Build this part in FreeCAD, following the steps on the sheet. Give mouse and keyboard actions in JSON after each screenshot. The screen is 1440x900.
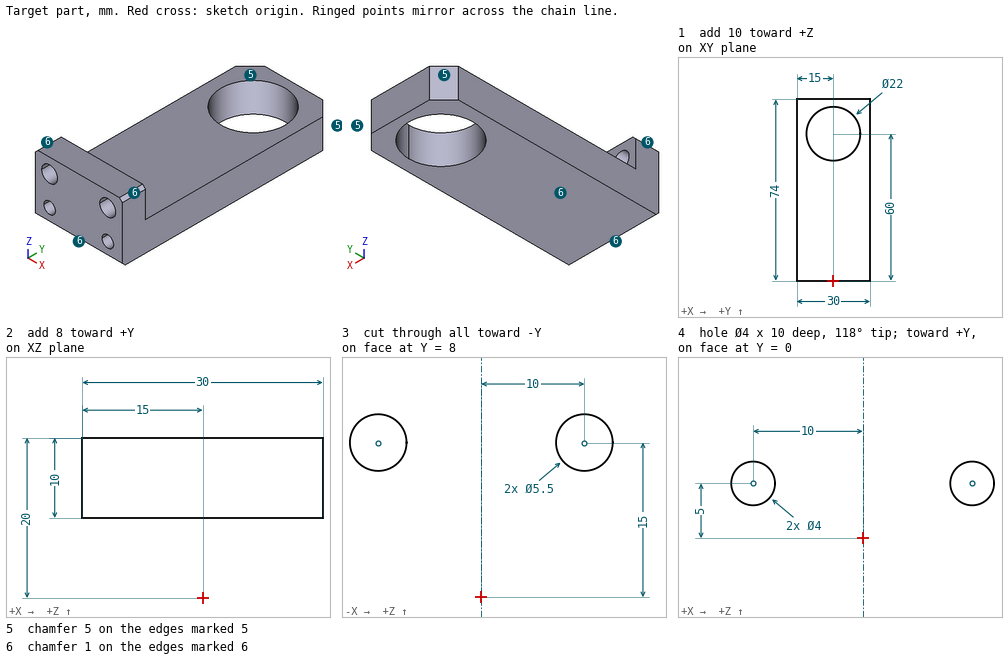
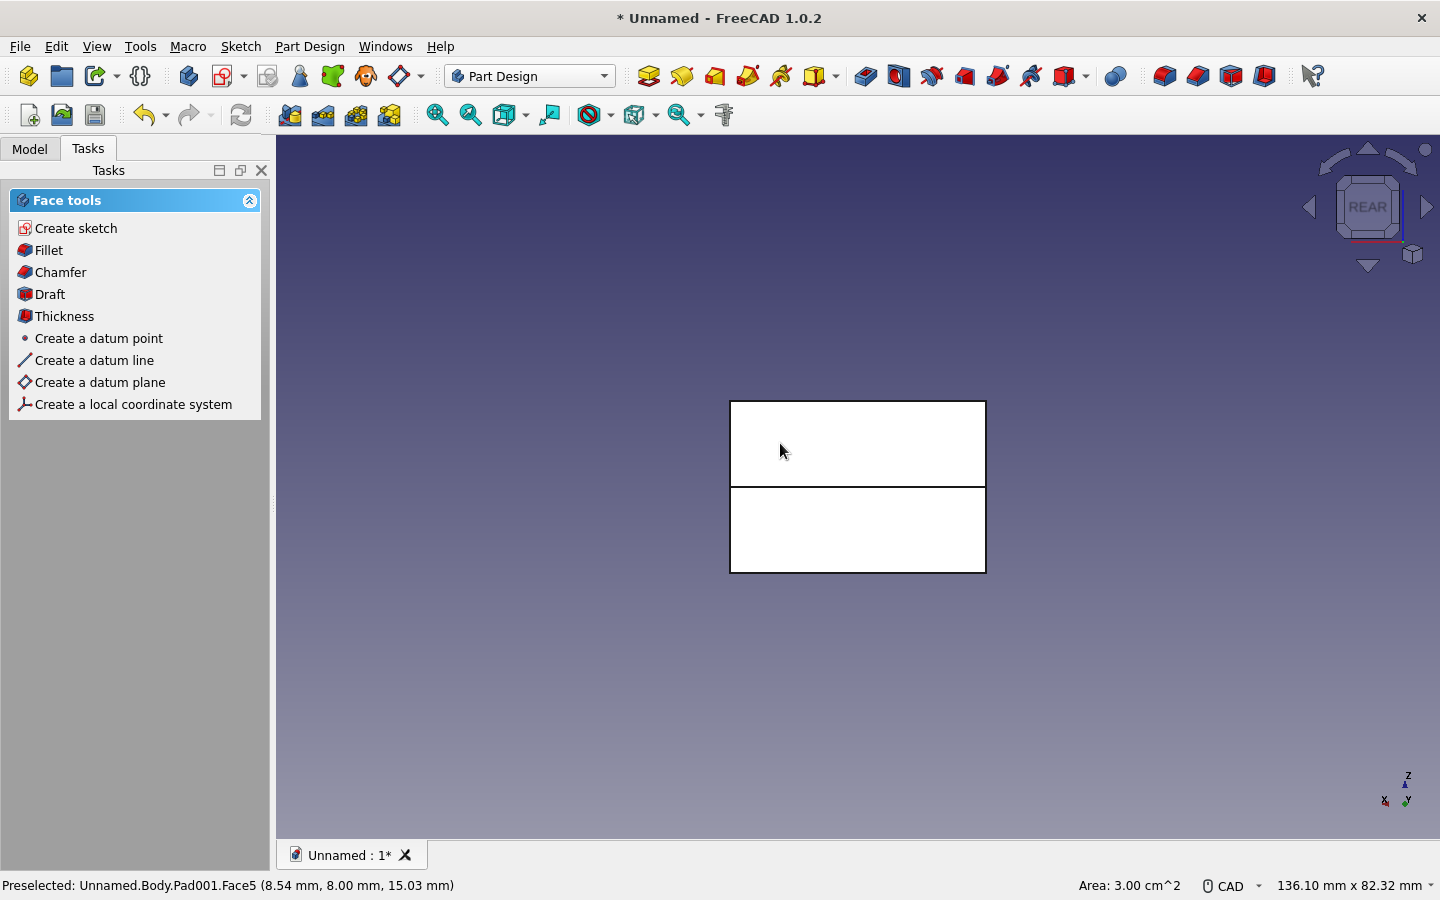
{"action": "left_click", "coordinate": [222, 76]}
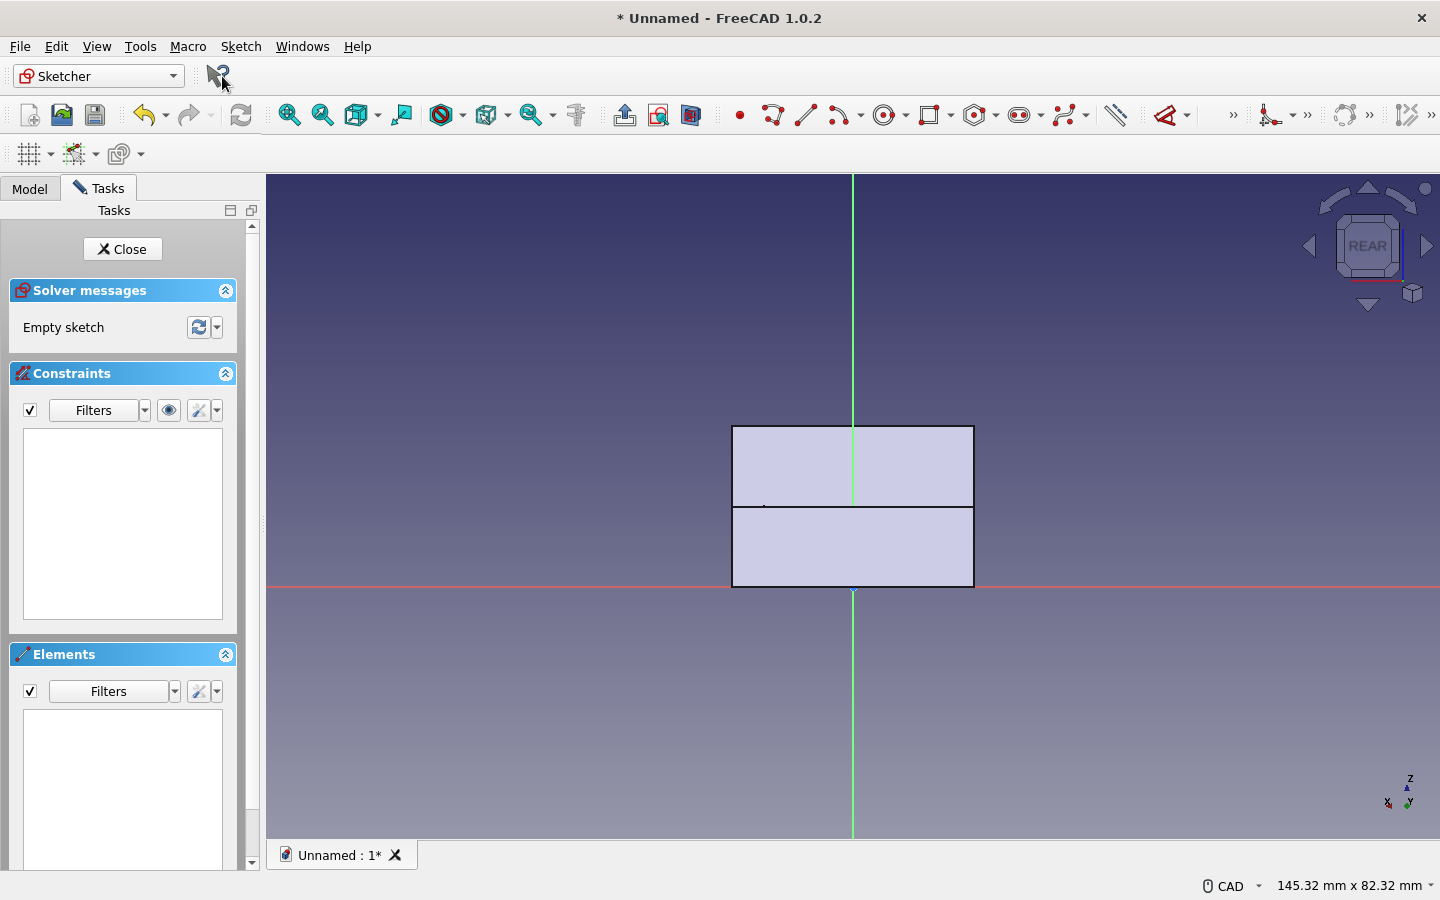
{"action": "left_click", "coordinate": [691, 116]}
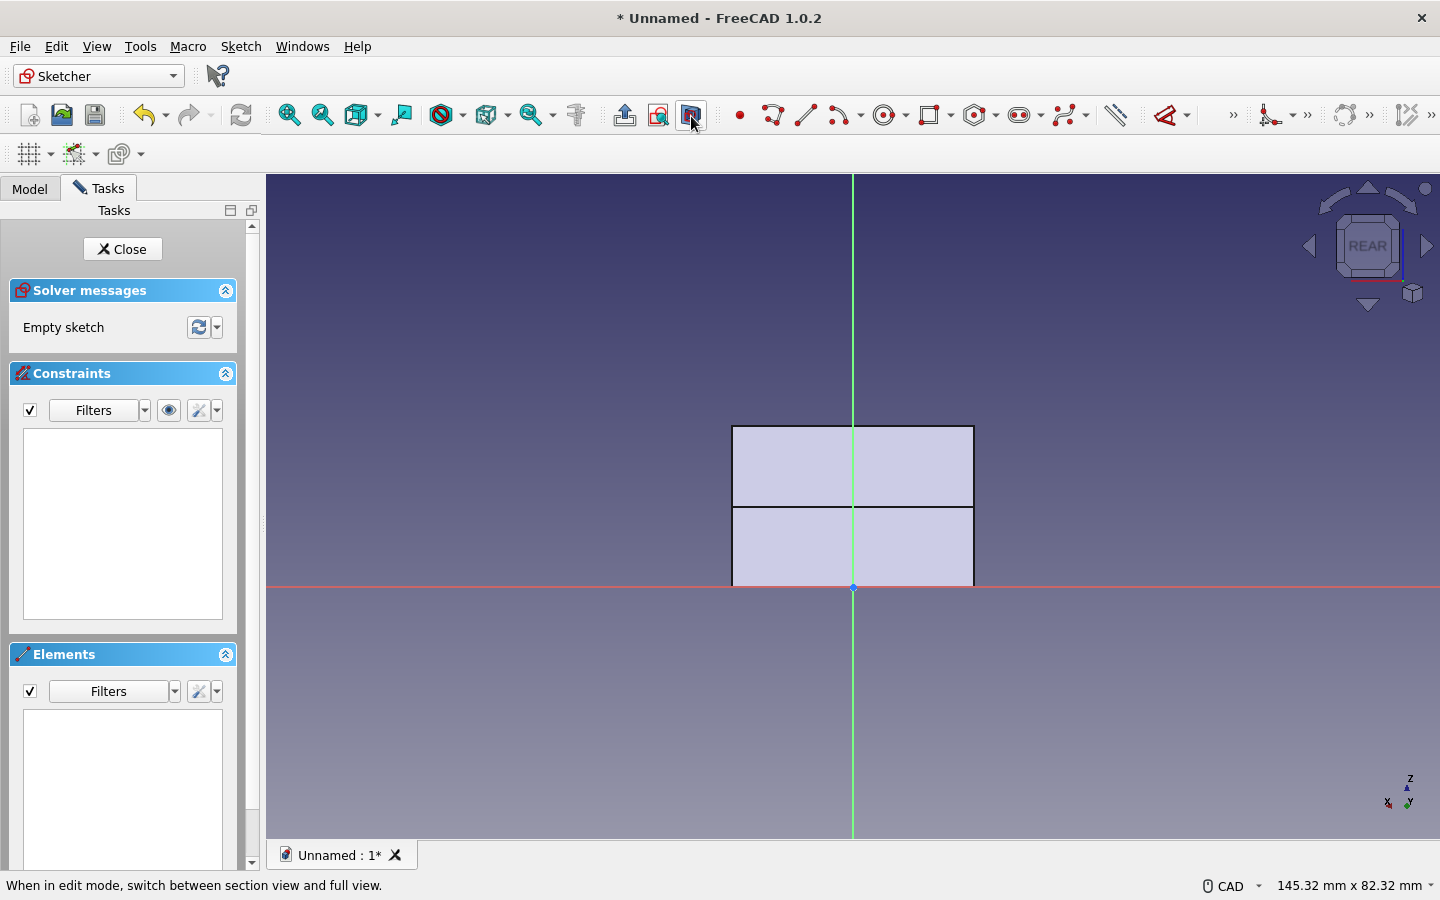
{"action": "scroll", "coordinate": [893, 521], "scroll_direction": "up", "scroll_amount": 5}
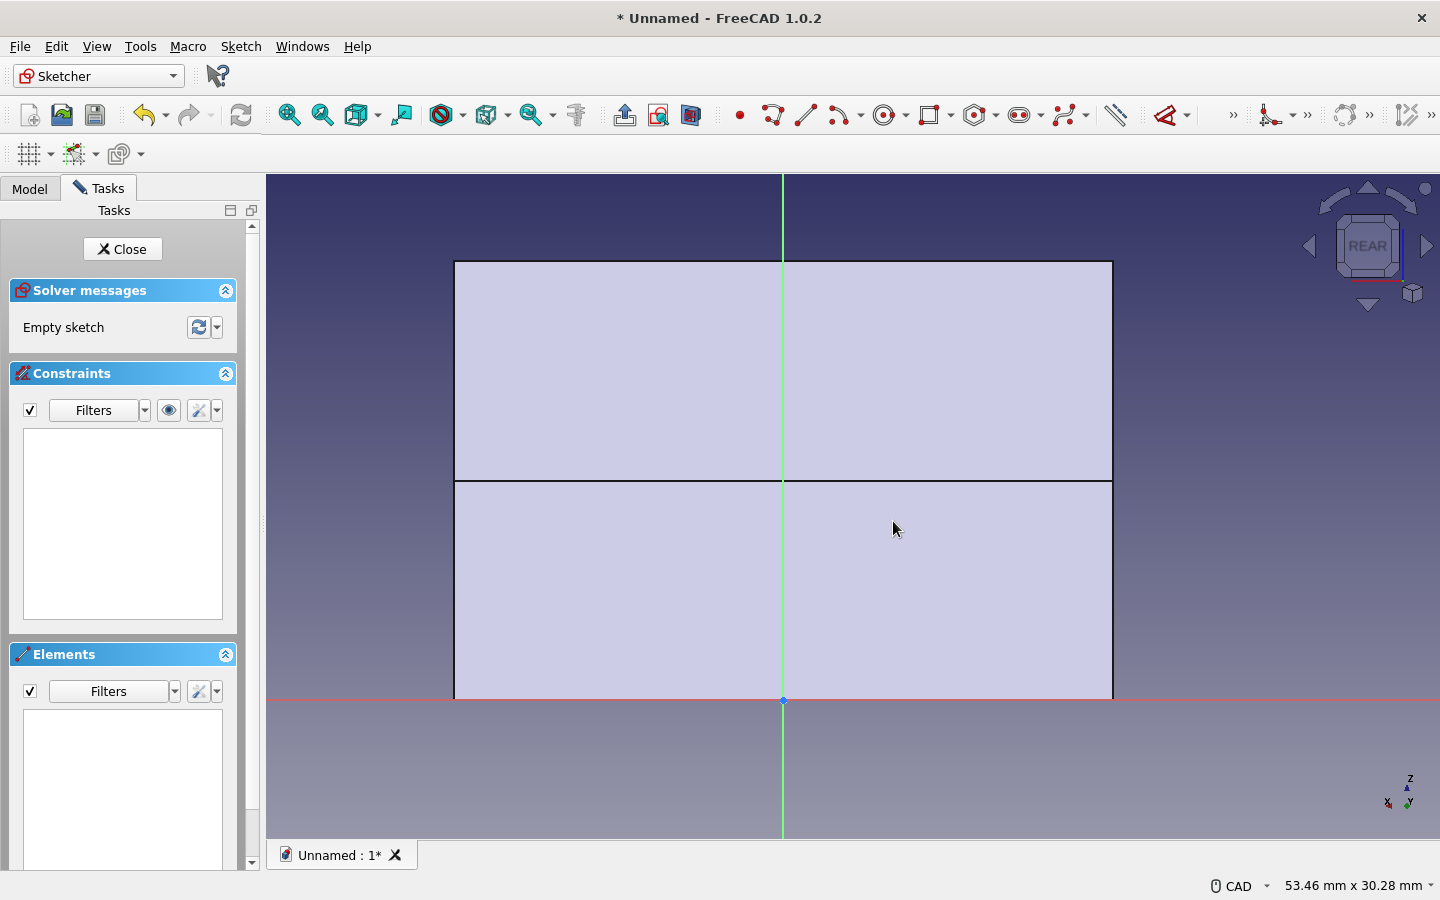
{"action": "left_click", "coordinate": [884, 116]}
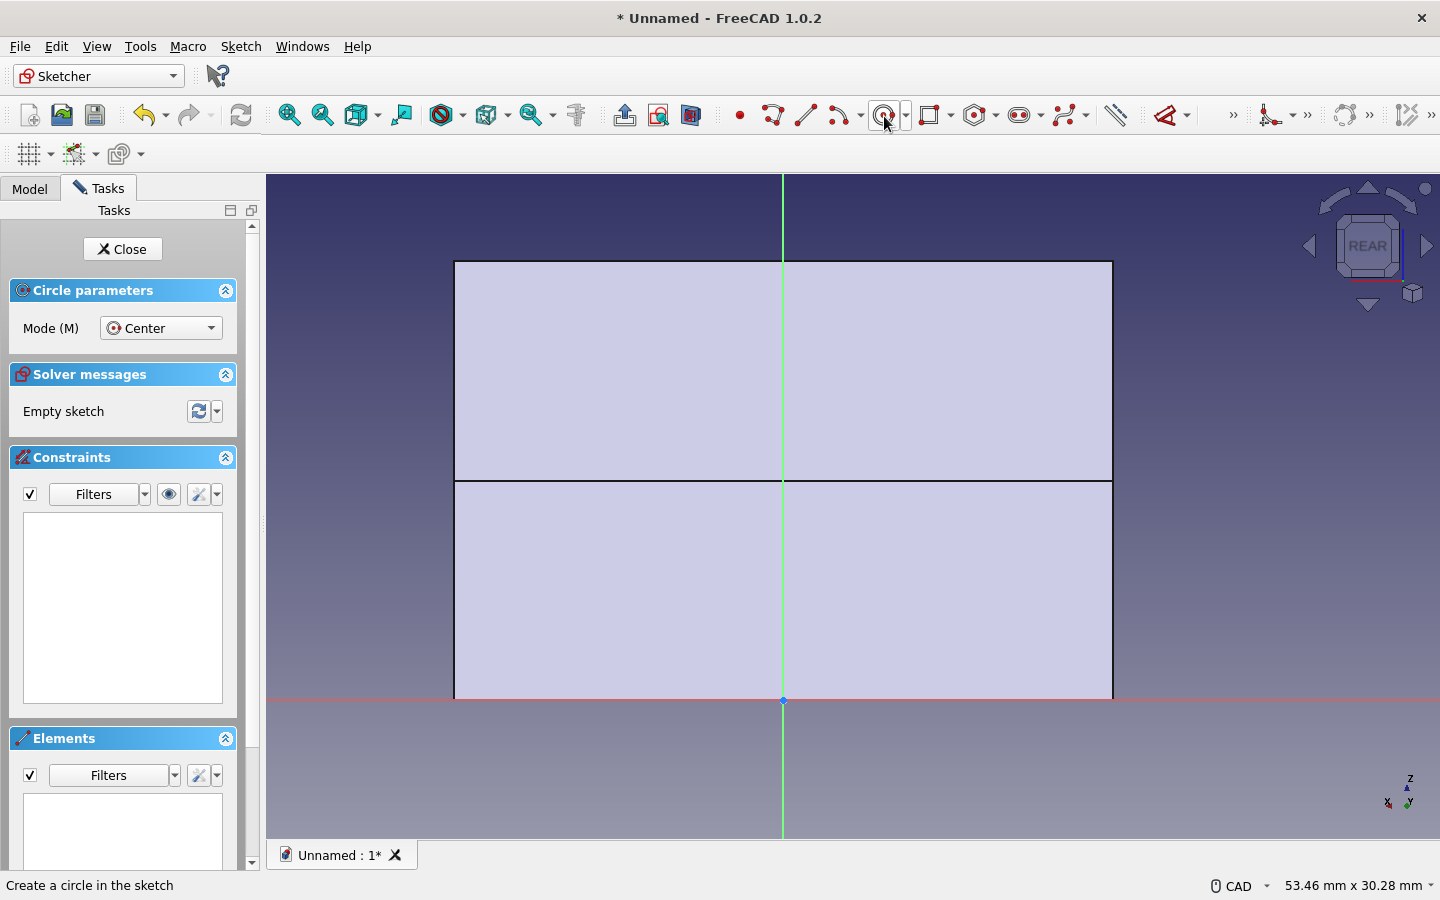
{"action": "left_click", "coordinate": [1003, 371]}
{"action": "left_click", "coordinate": [1046, 328]}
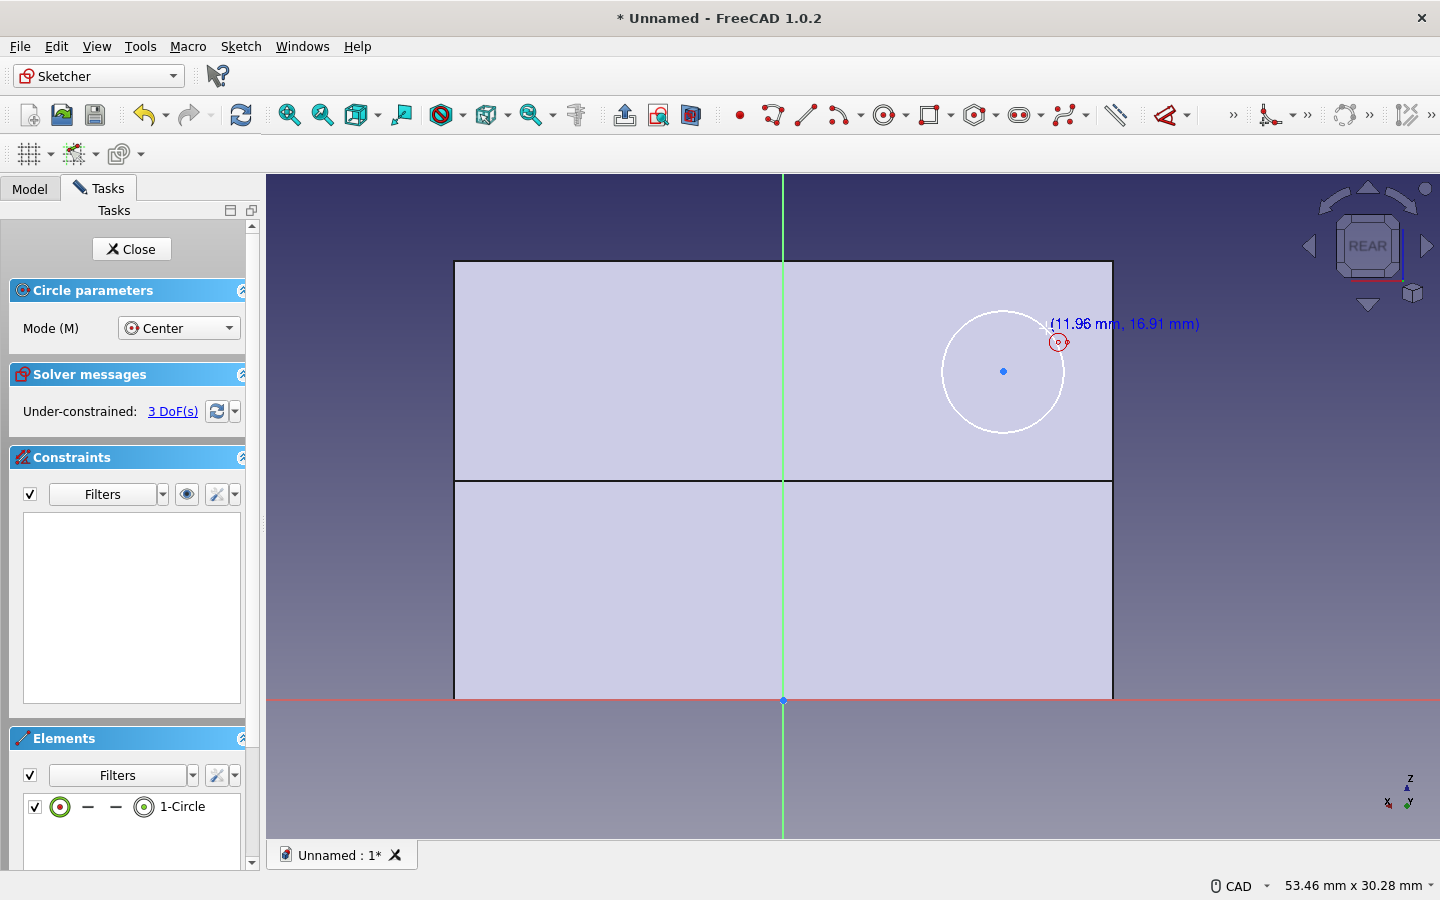
{"action": "left_click", "coordinate": [564, 371]}
{"action": "left_click", "coordinate": [606, 328]}
{"action": "key", "text": "Escape"}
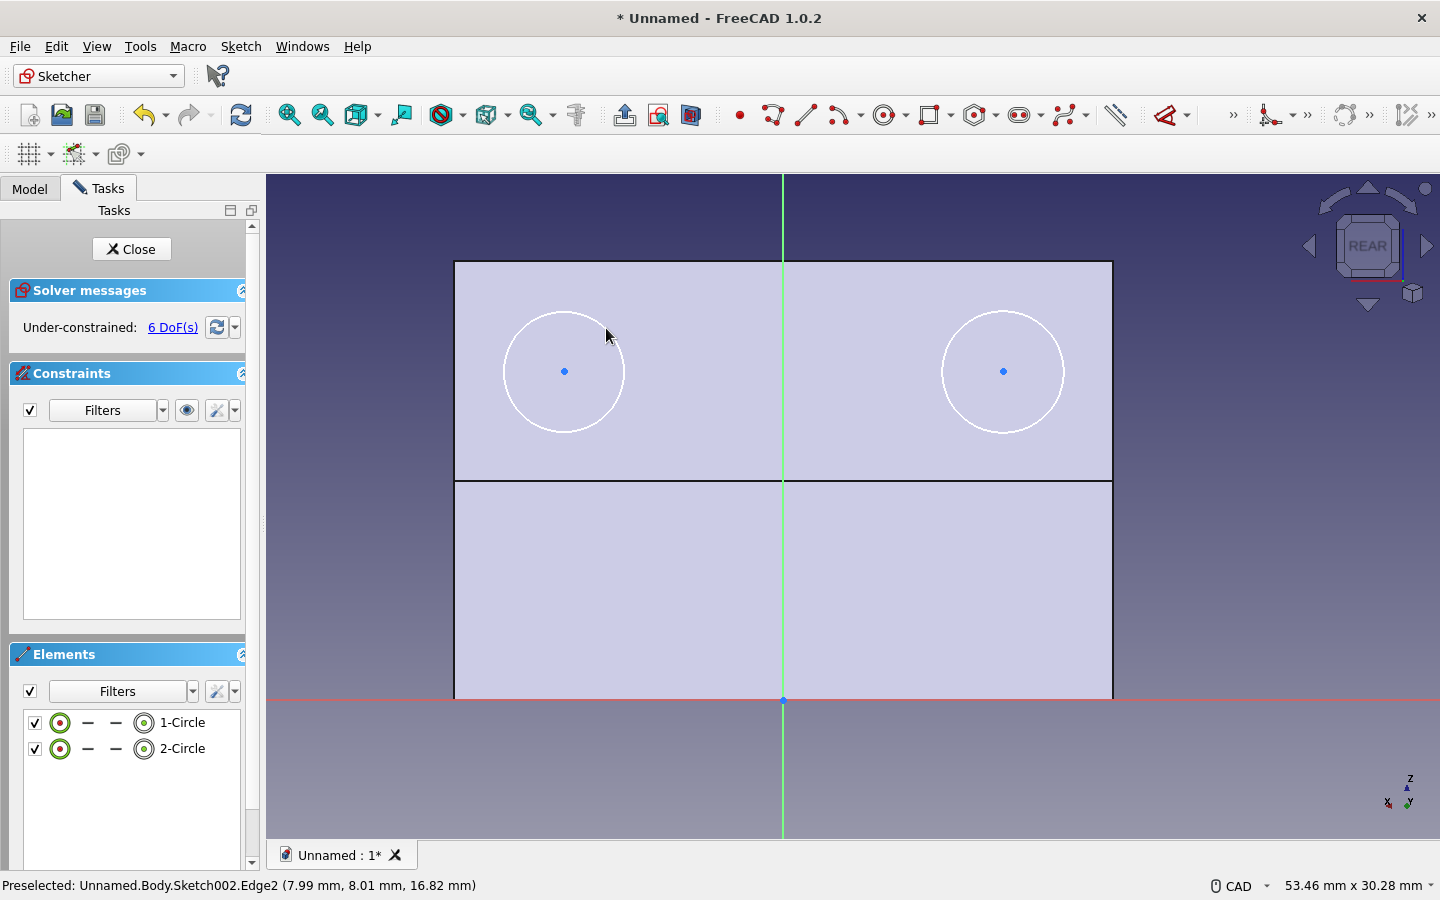
{"action": "left_click", "coordinate": [1046, 329]}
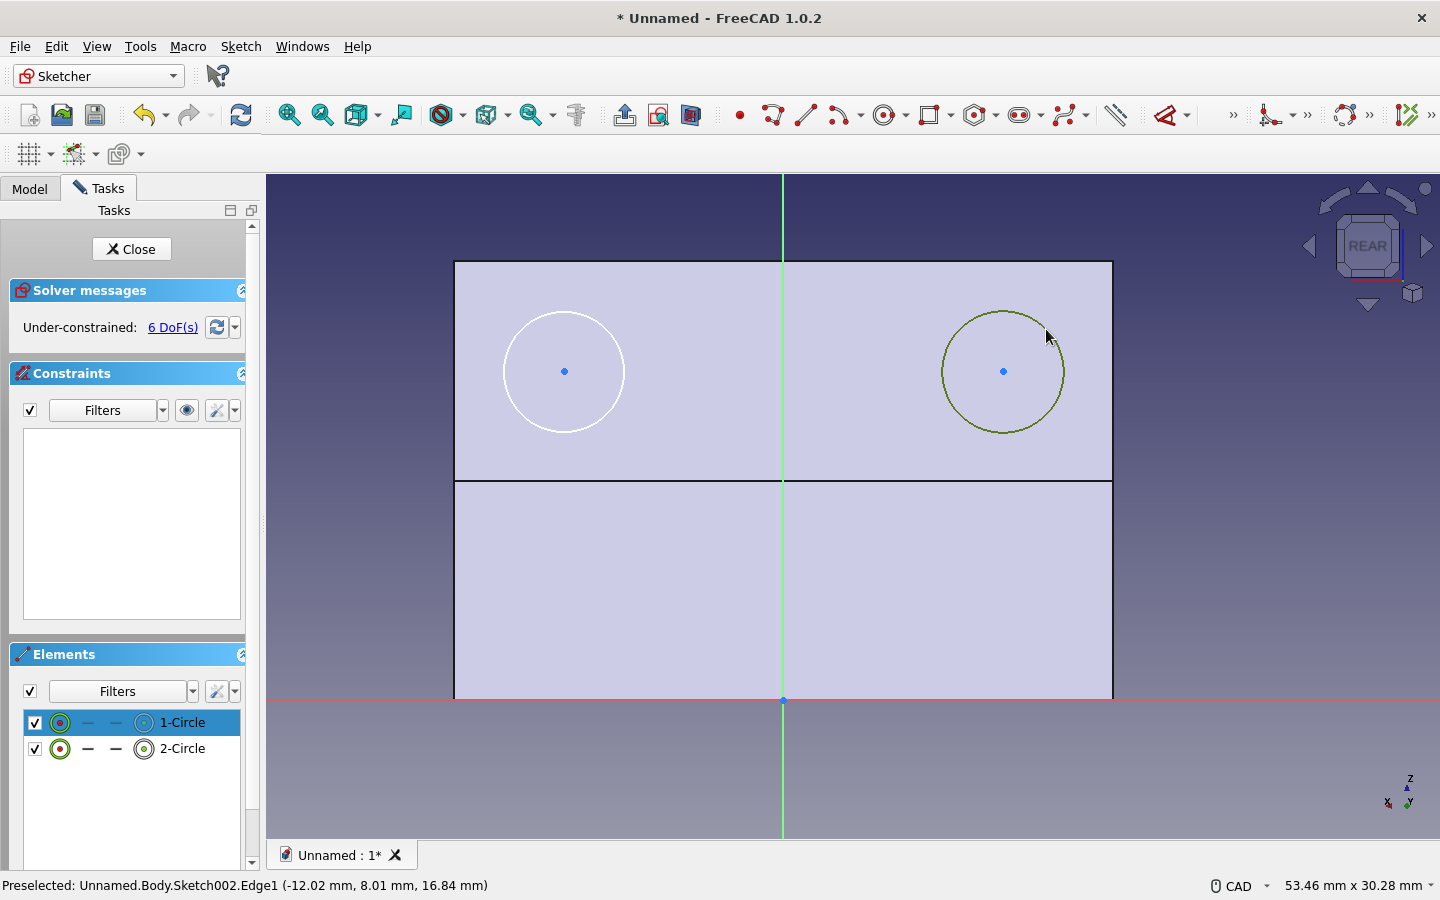
{"action": "left_click", "coordinate": [606, 329]}